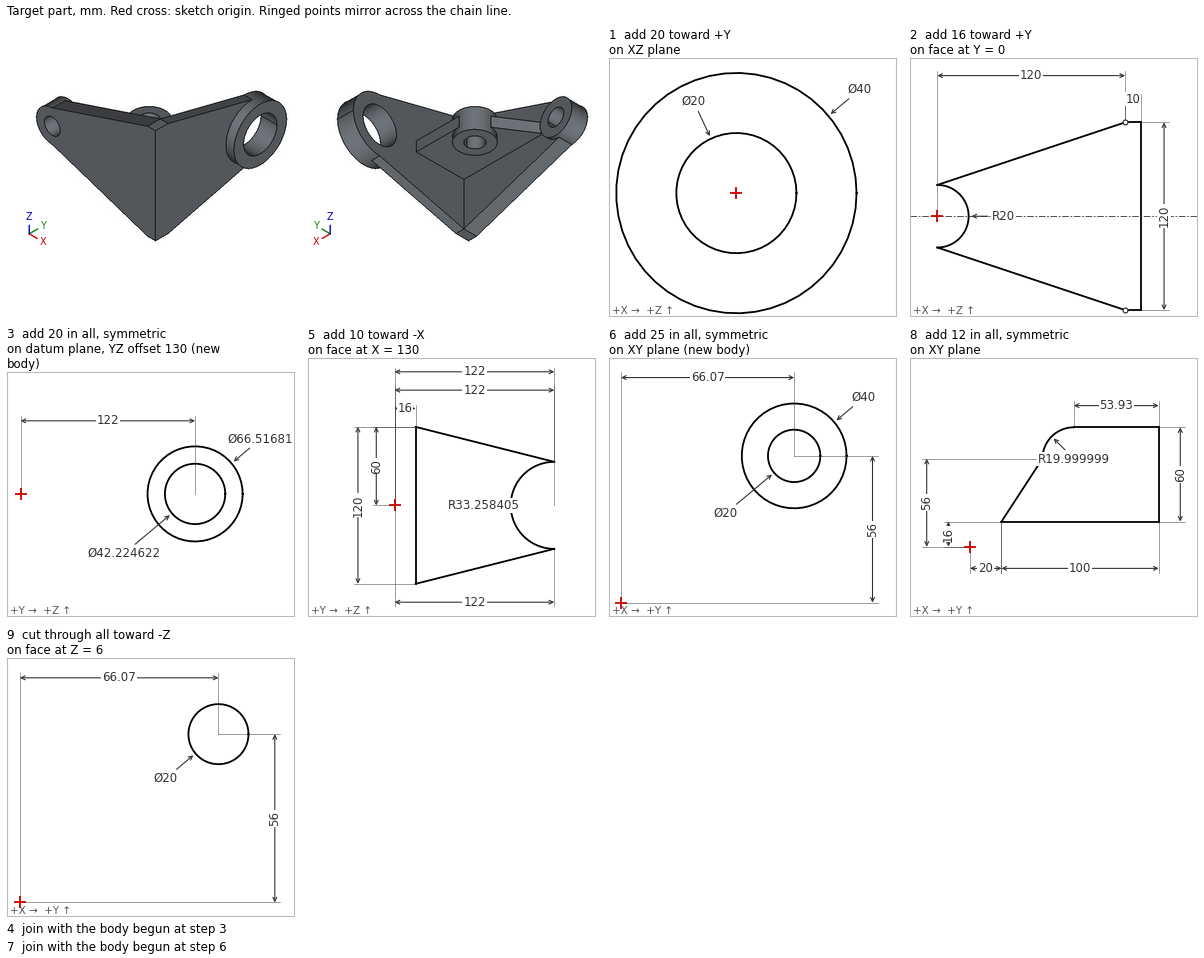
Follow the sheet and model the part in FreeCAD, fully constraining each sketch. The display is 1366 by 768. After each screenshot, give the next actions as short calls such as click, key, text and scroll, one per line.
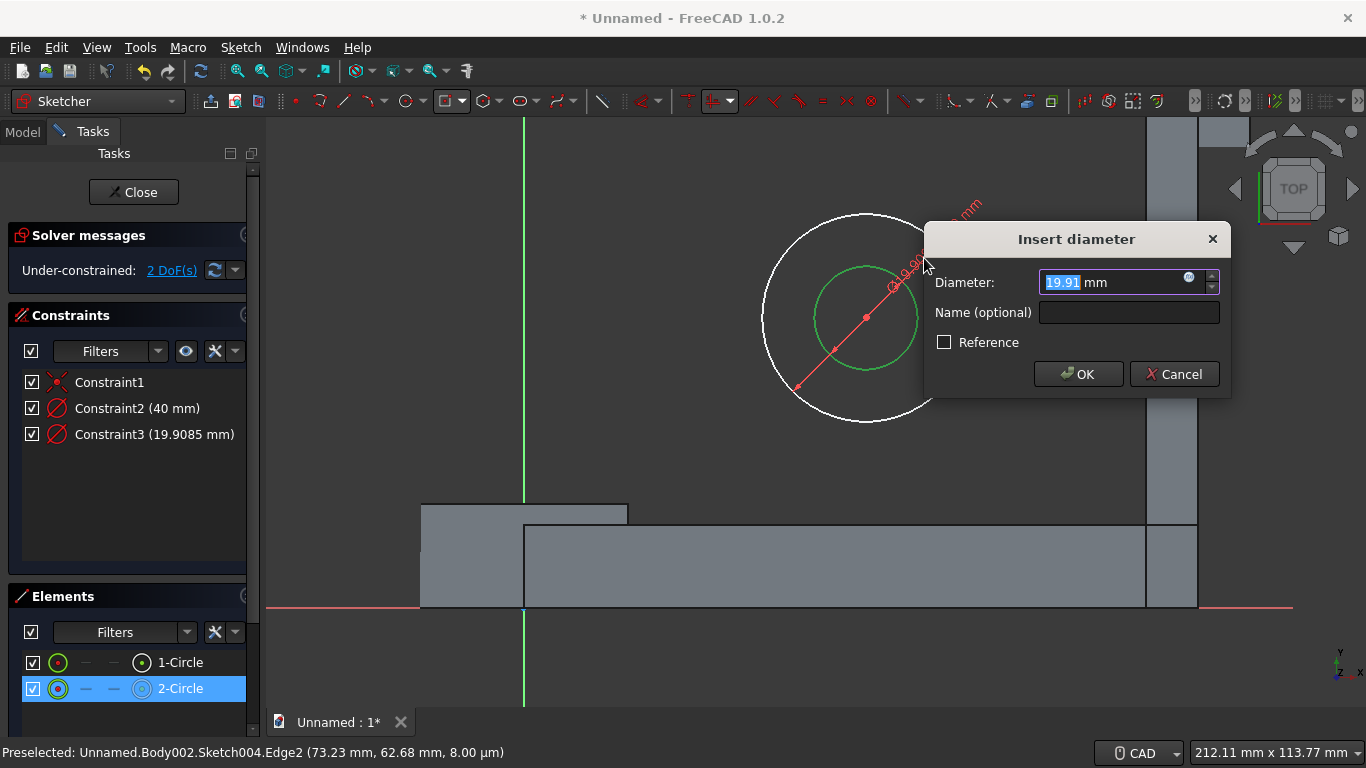
text(20)
key(Return)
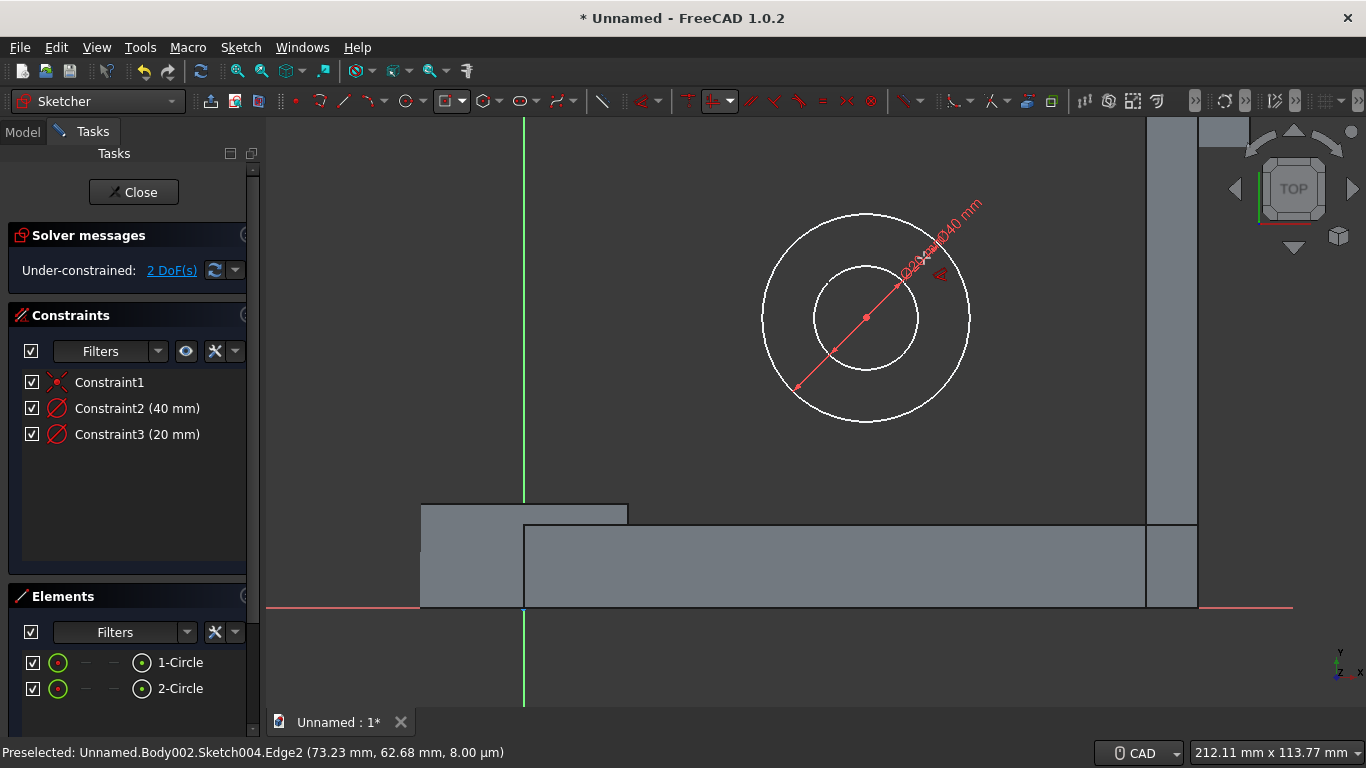
click(866, 318)
click(490, 463)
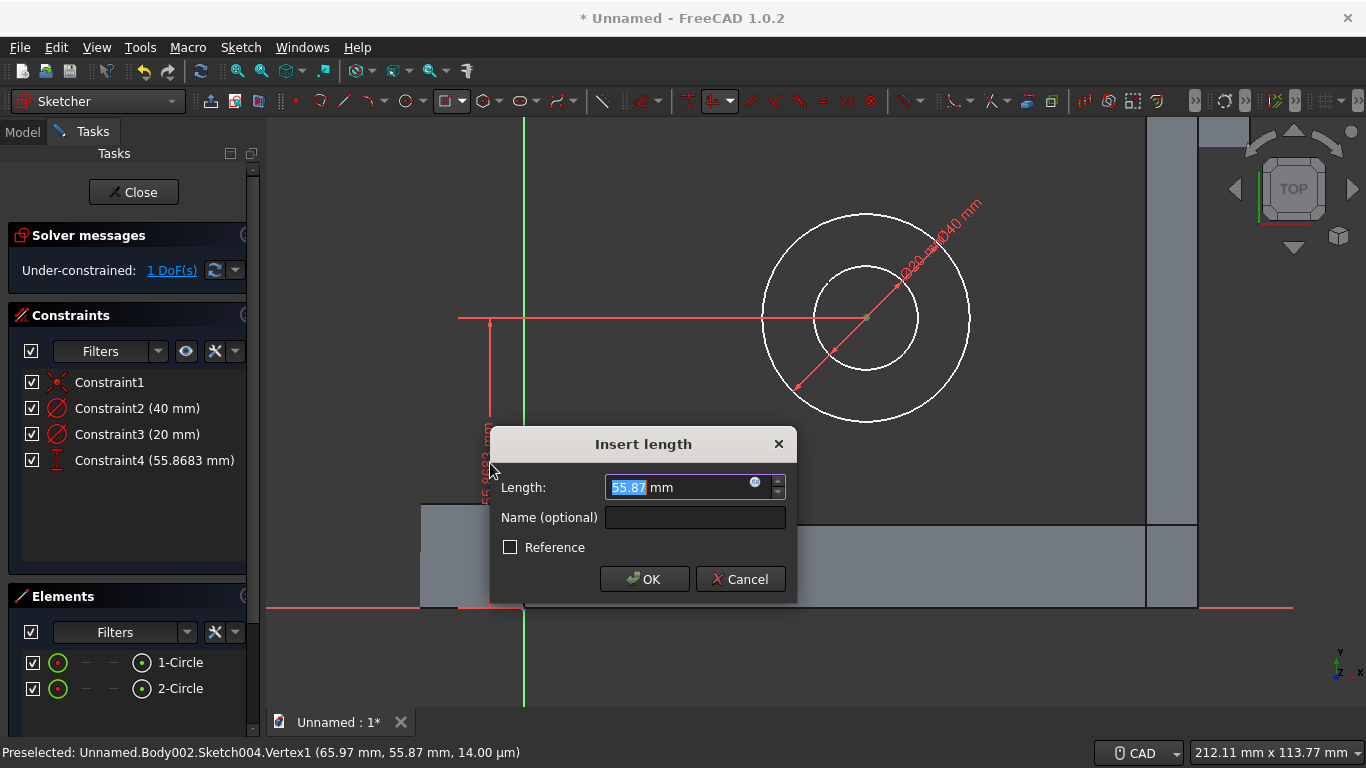
text(56)
key(Return)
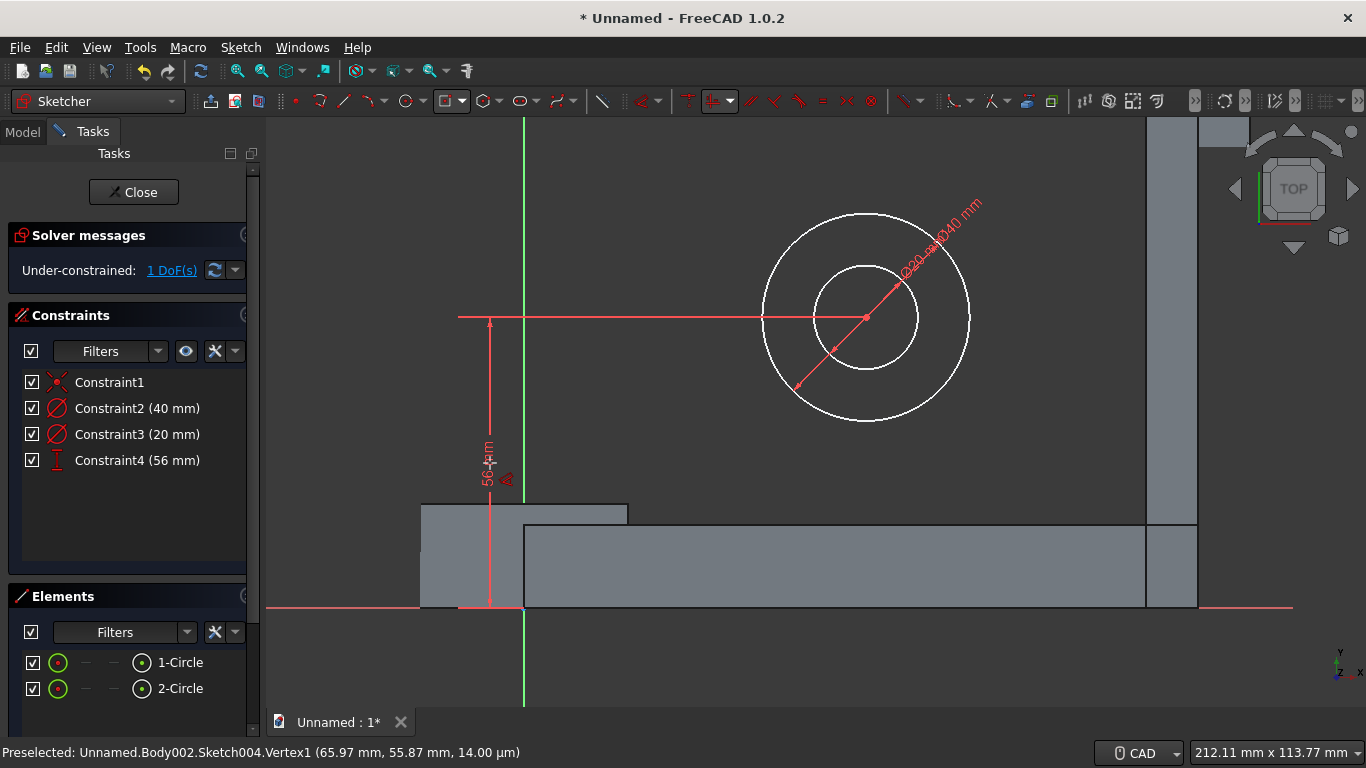
click(866, 317)
click(695, 642)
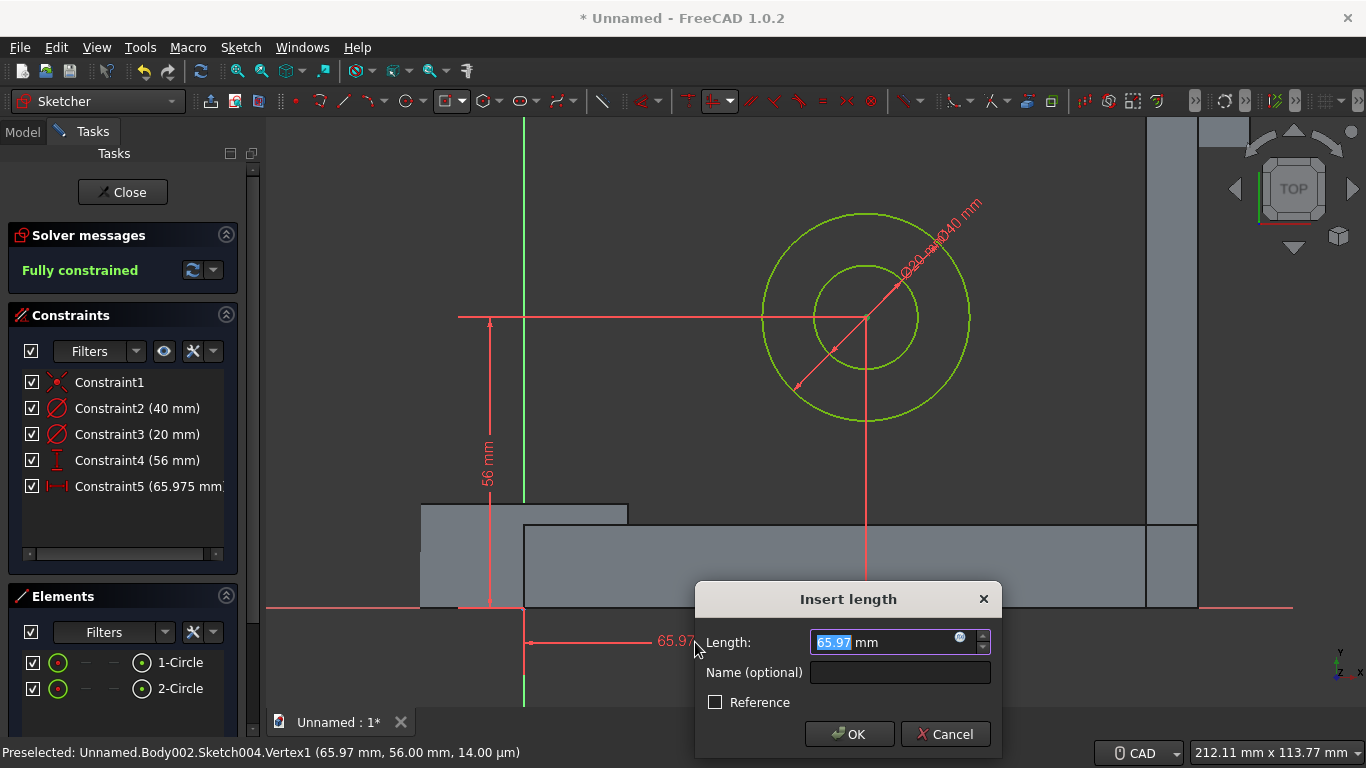
text(66.07)
key(Return)
key(Escape)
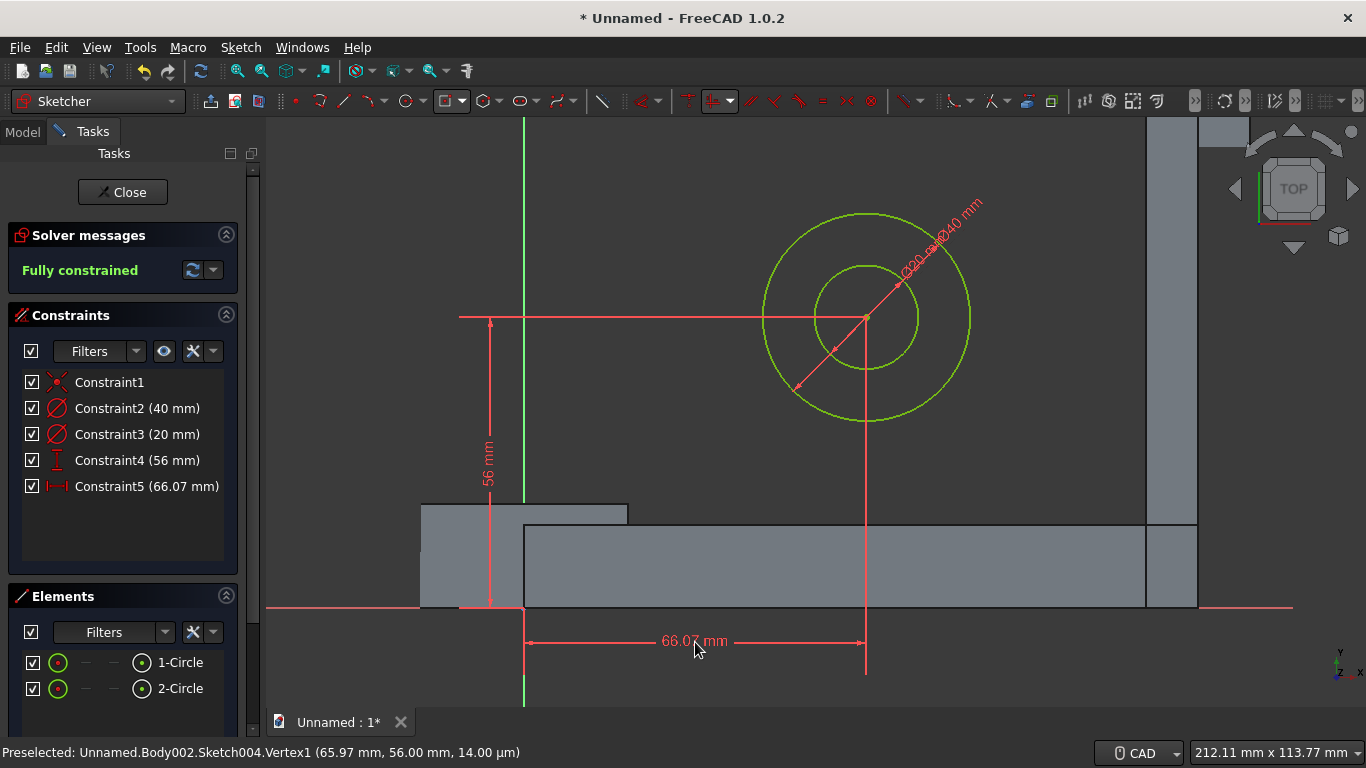
click(123, 192)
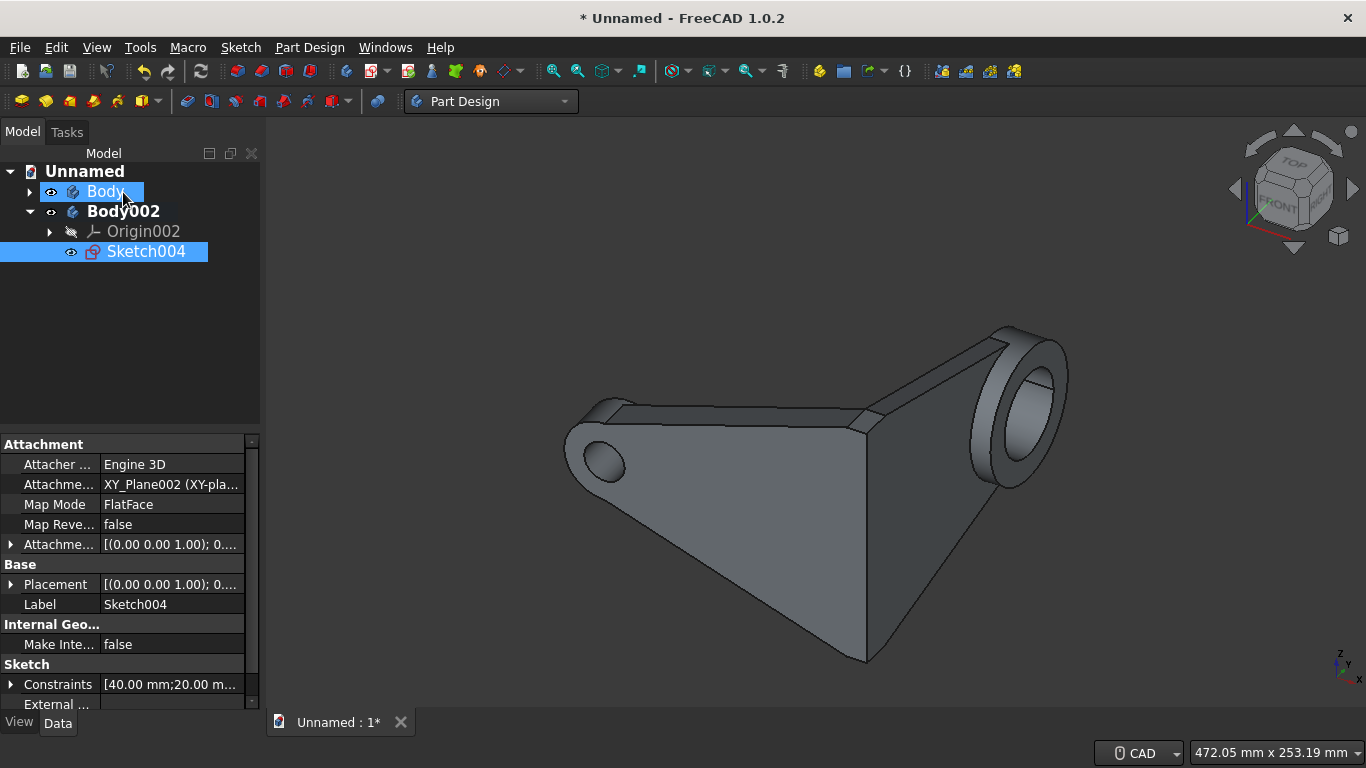
click(22, 102)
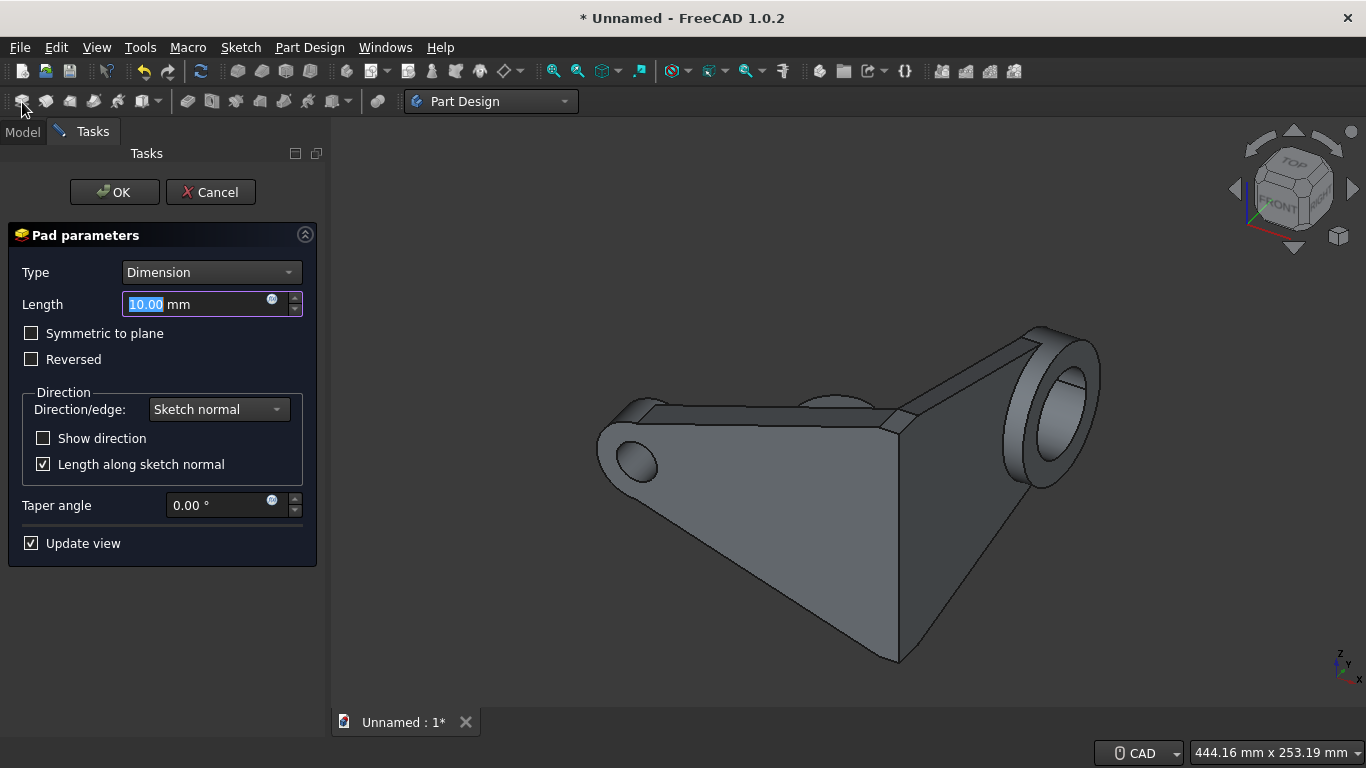
text(25)
key(Tab)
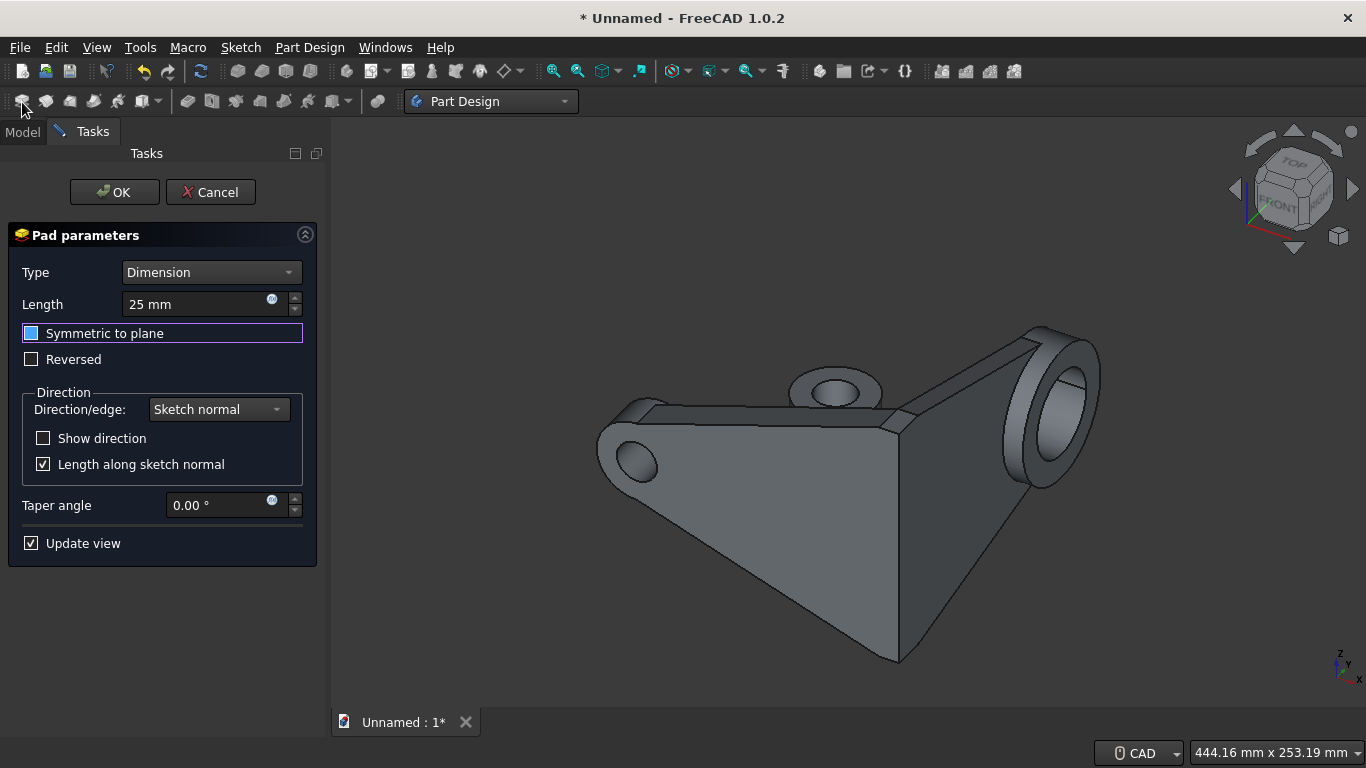
click(30, 333)